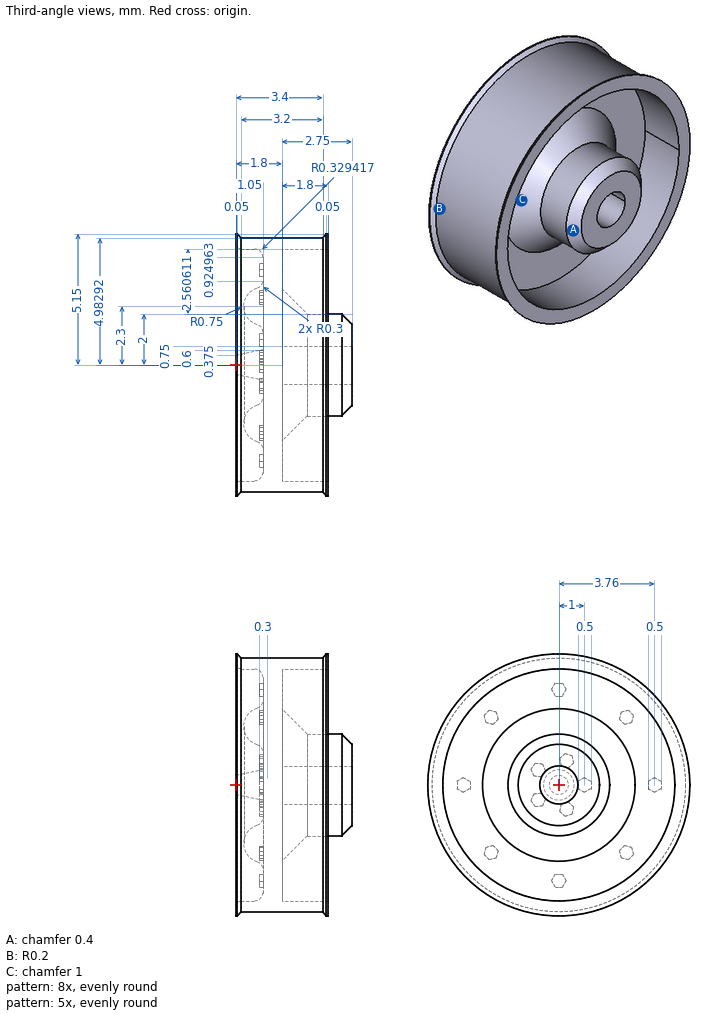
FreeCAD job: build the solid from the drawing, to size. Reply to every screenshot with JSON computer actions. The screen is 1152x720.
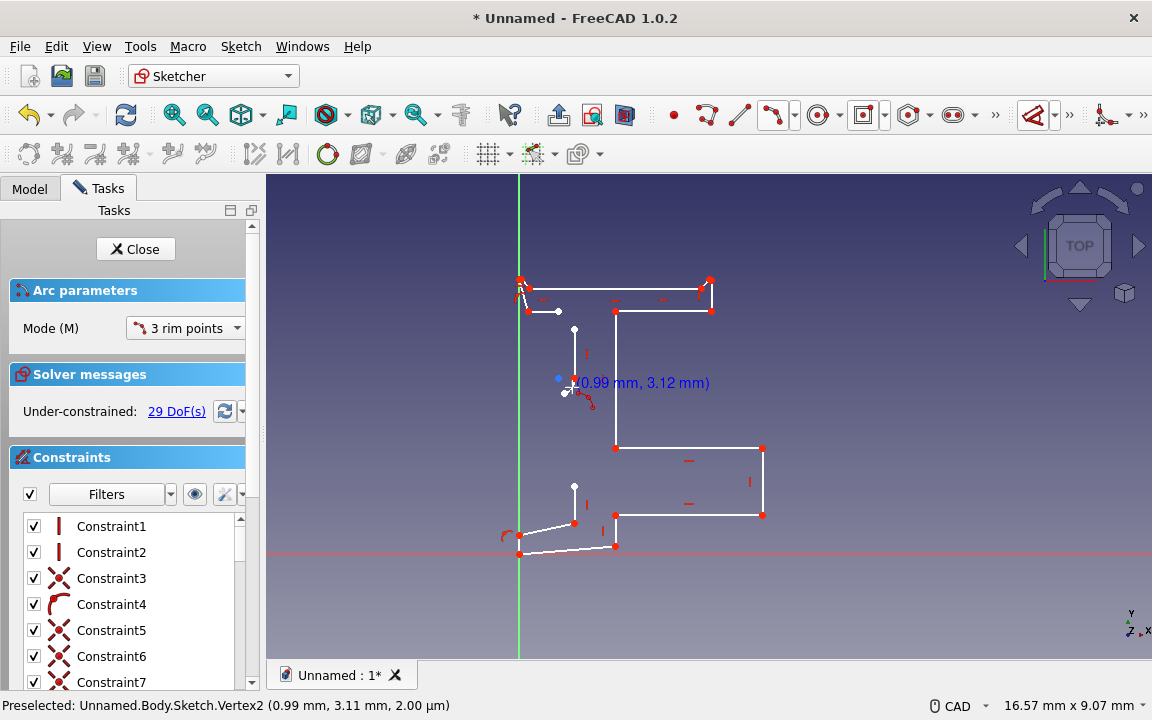
{"action": "left_click", "coordinate": [564, 394]}
{"action": "left_click", "coordinate": [564, 470]}
{"action": "left_click", "coordinate": [535, 432]}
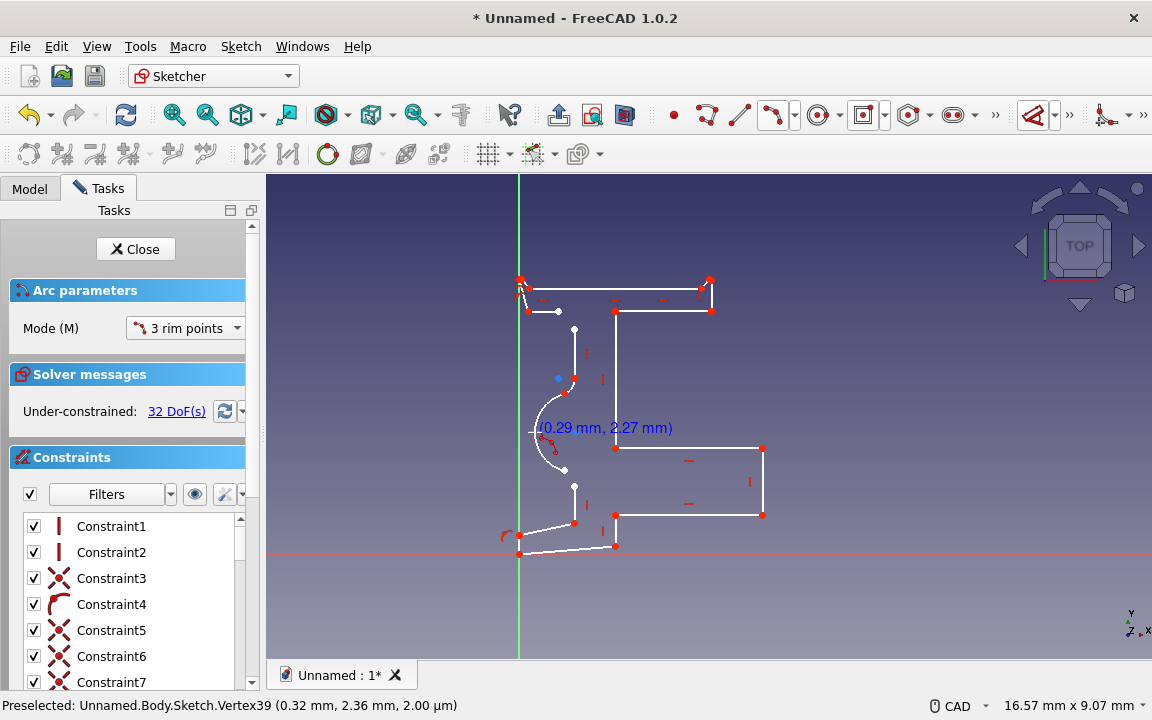
{"action": "left_click", "coordinate": [564, 471]}
{"action": "left_click", "coordinate": [575, 486]}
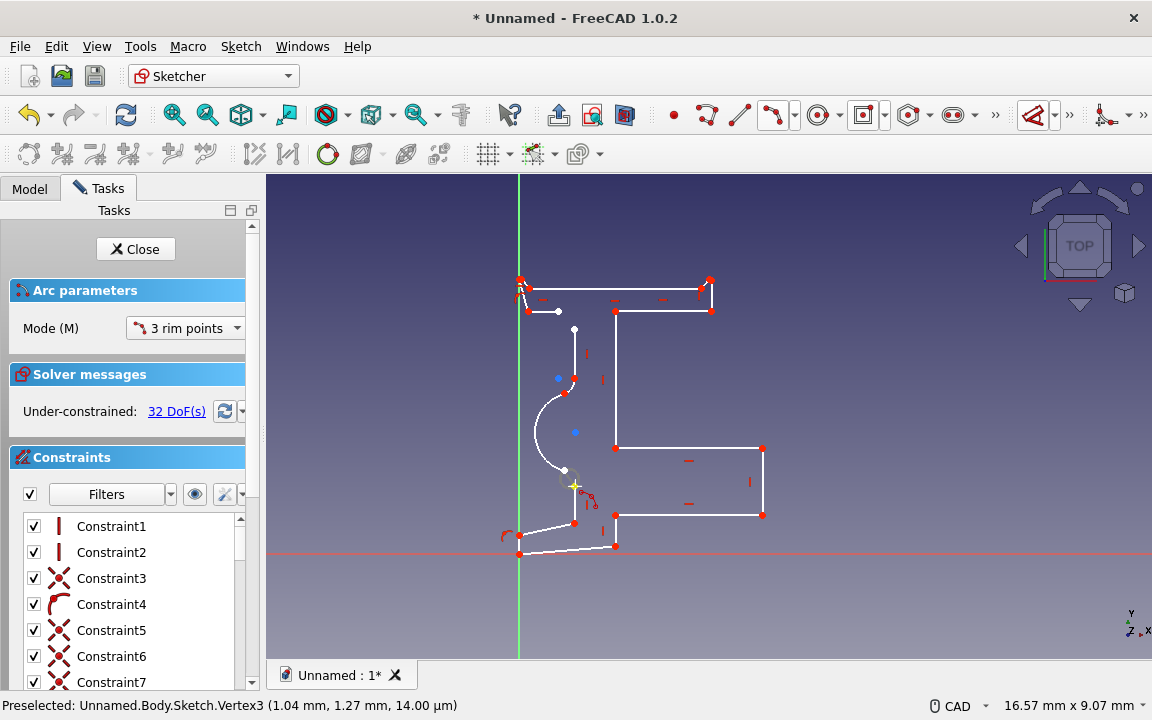
{"action": "scroll", "coordinate": [572, 476], "scroll_direction": "up", "scroll_amount": 9}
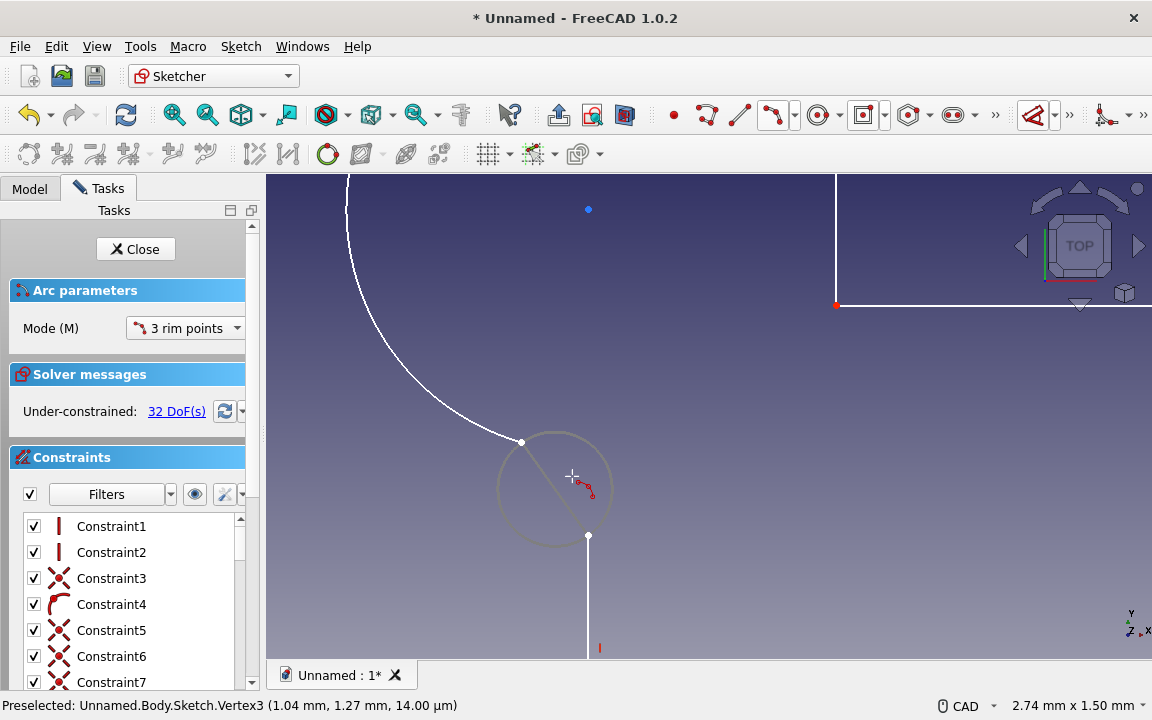
{"action": "left_click", "coordinate": [572, 471]}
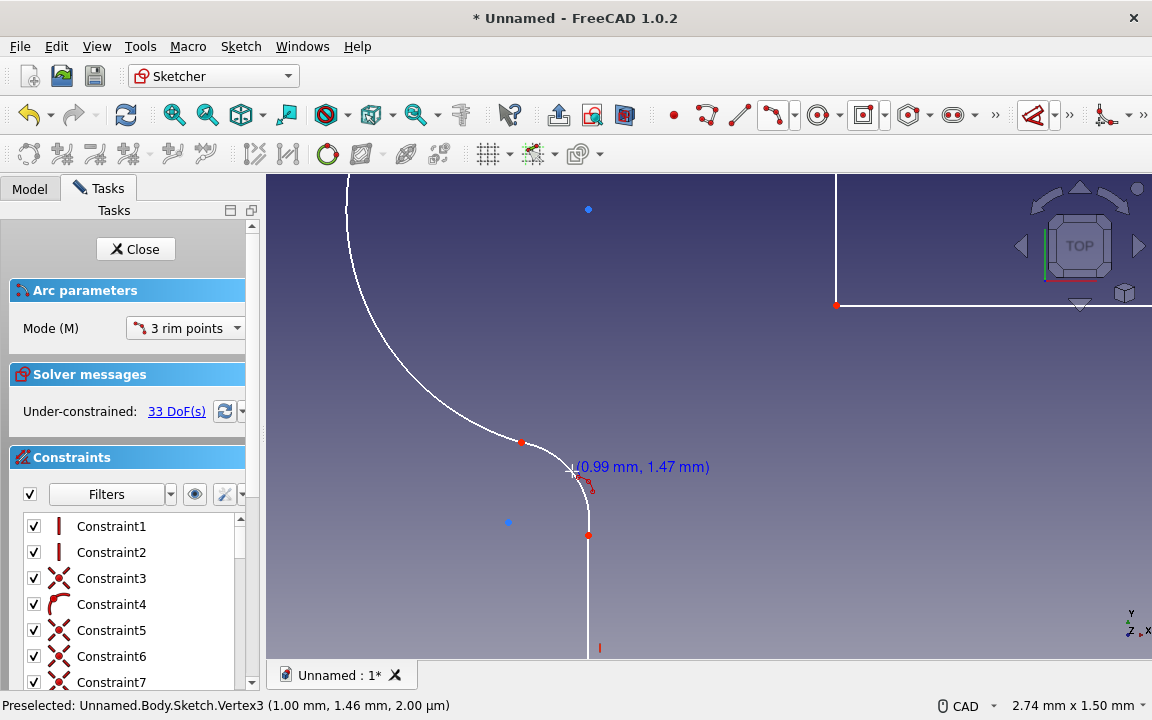
{"action": "scroll", "coordinate": [572, 476], "scroll_direction": "down", "scroll_amount": 9}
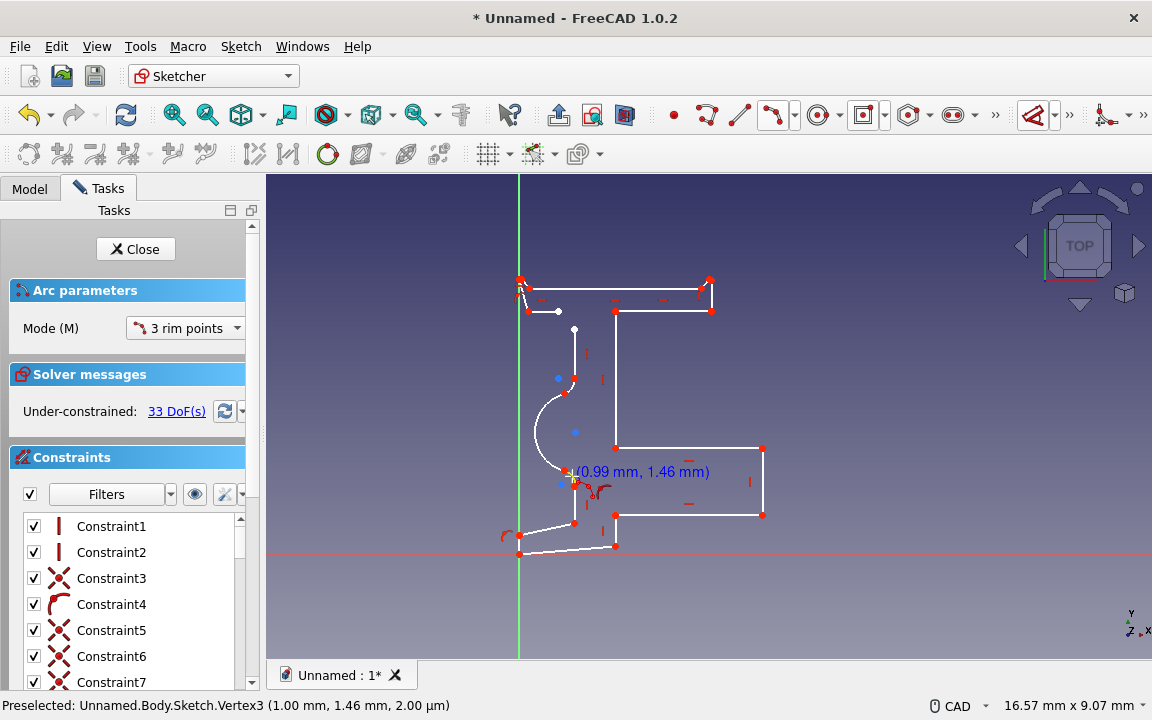
{"action": "left_click", "coordinate": [558, 312]}
{"action": "left_click", "coordinate": [575, 329]}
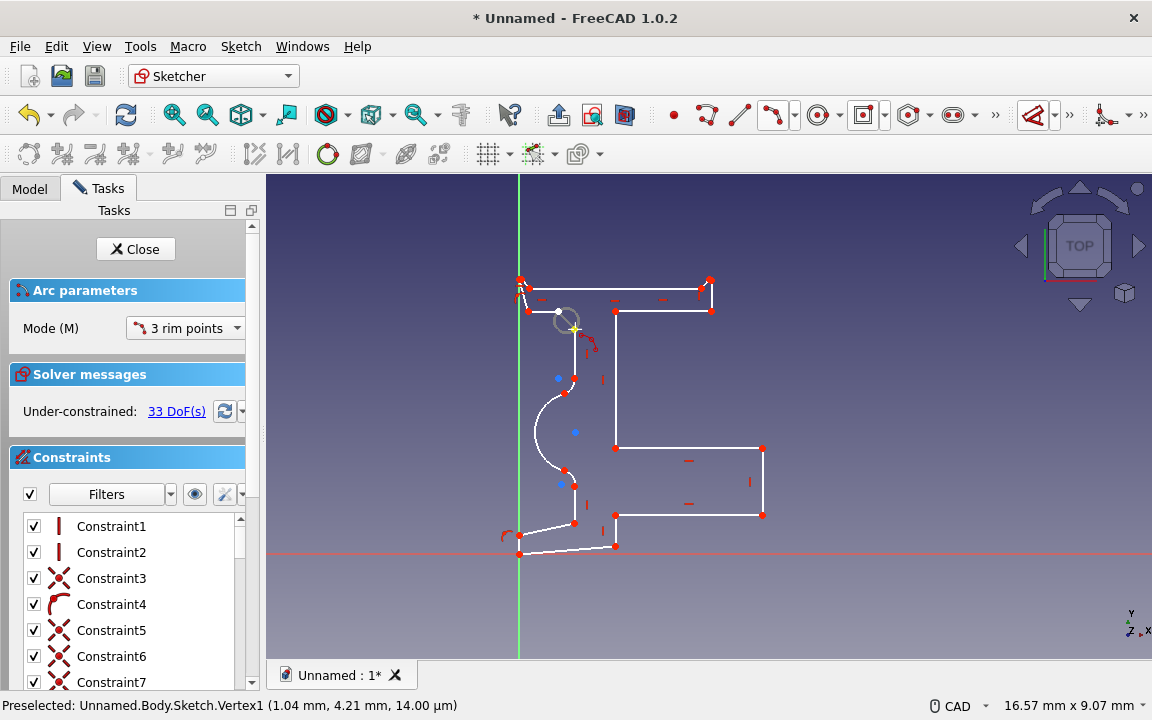
{"action": "scroll", "coordinate": [570, 316], "scroll_direction": "up", "scroll_amount": 6}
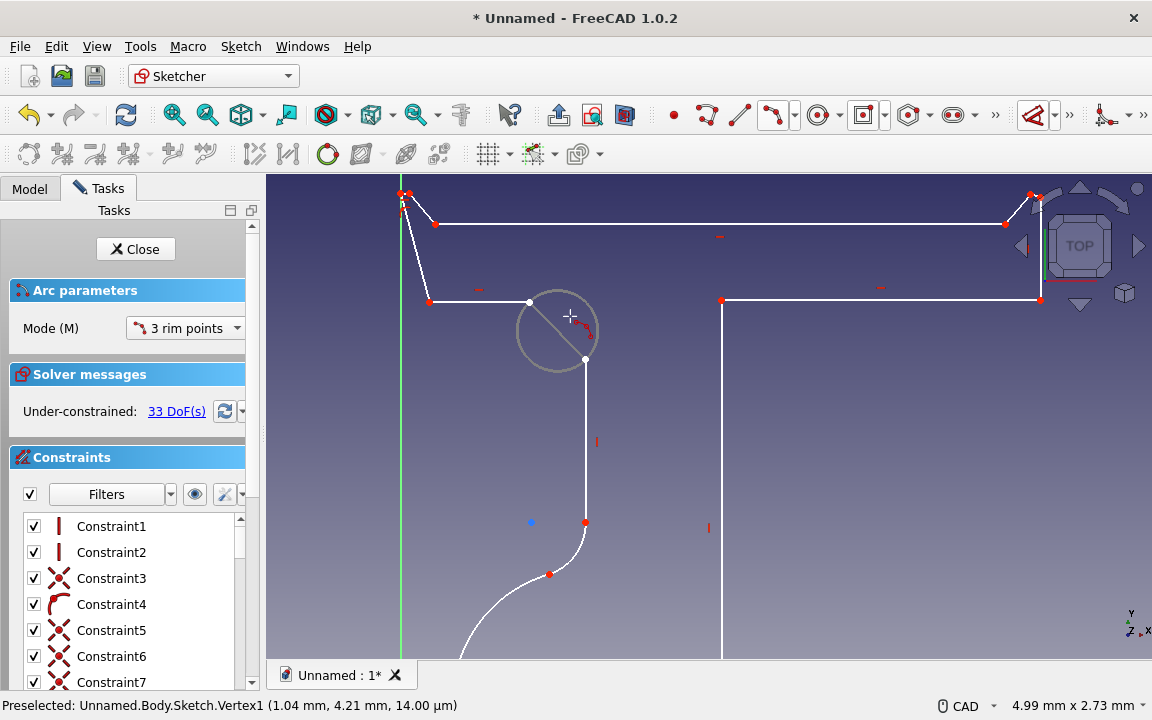
{"action": "left_click", "coordinate": [570, 315]}
{"action": "key", "text": "Escape"}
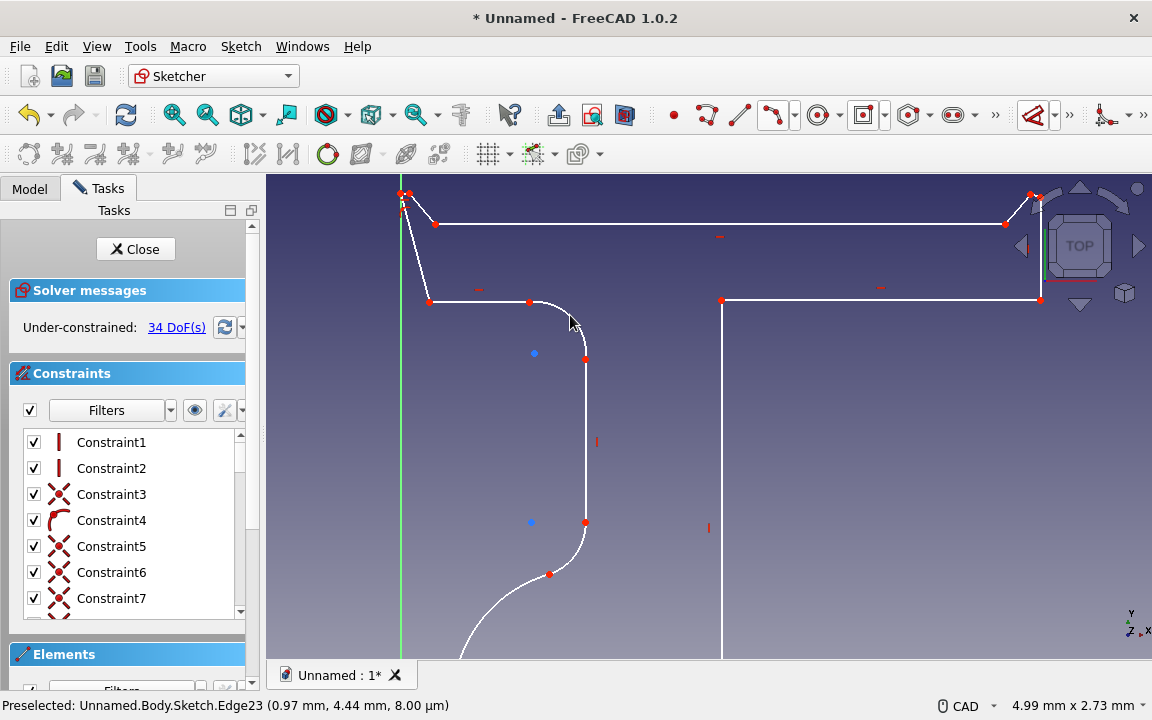
{"action": "left_click", "coordinate": [586, 409]}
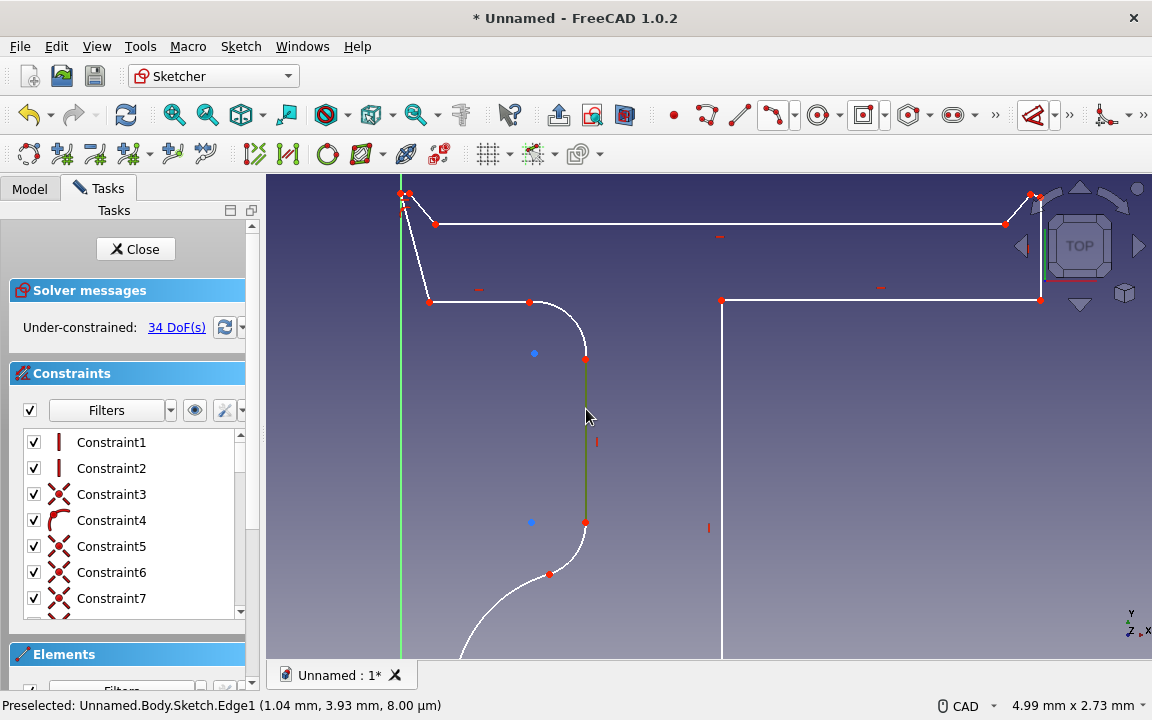
{"action": "left_click", "coordinate": [567, 564]}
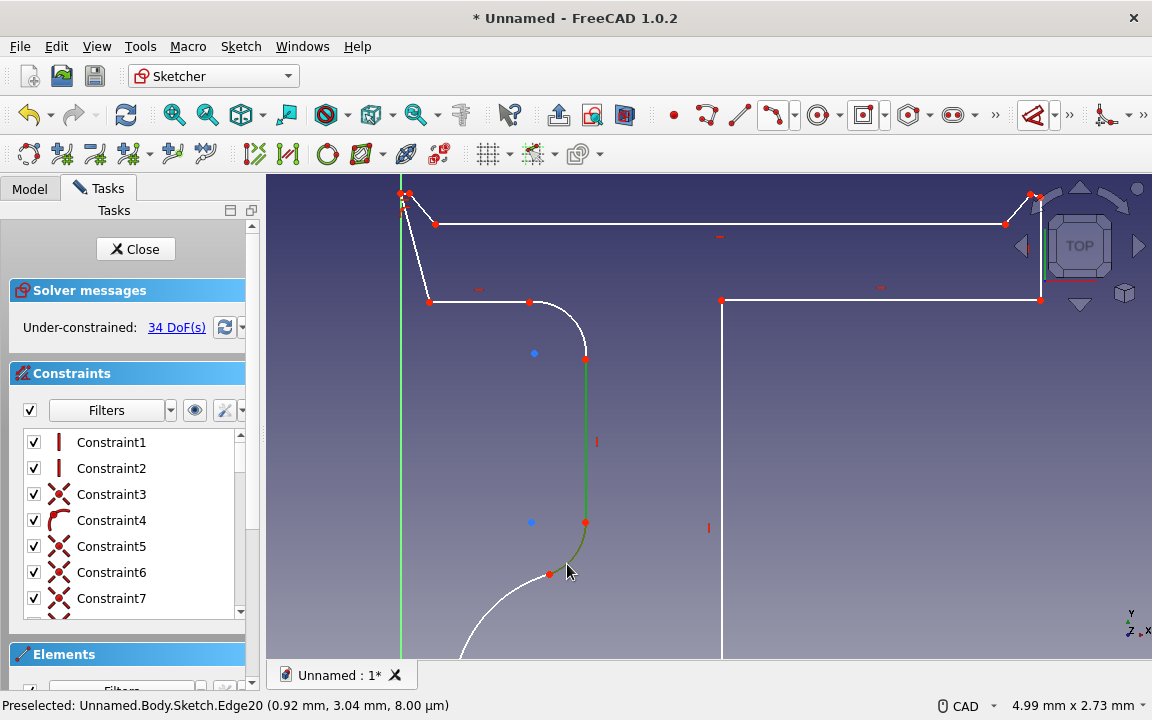
{"action": "key", "text": "t"}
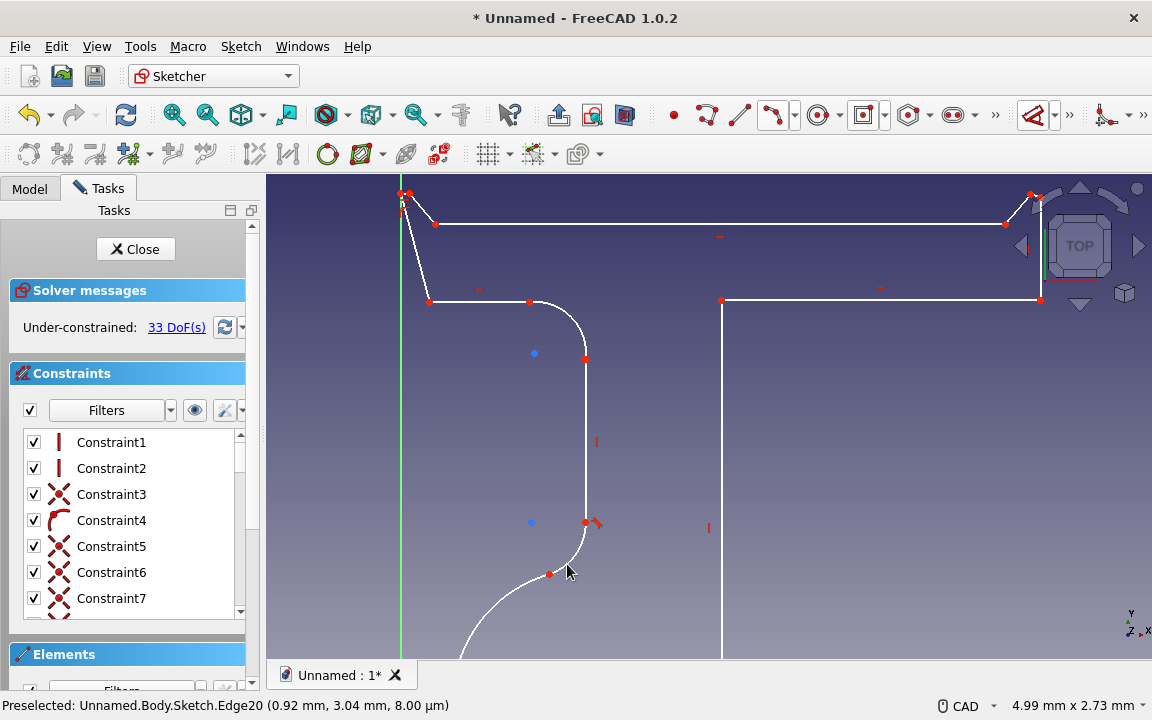
{"action": "left_click", "coordinate": [586, 409]}